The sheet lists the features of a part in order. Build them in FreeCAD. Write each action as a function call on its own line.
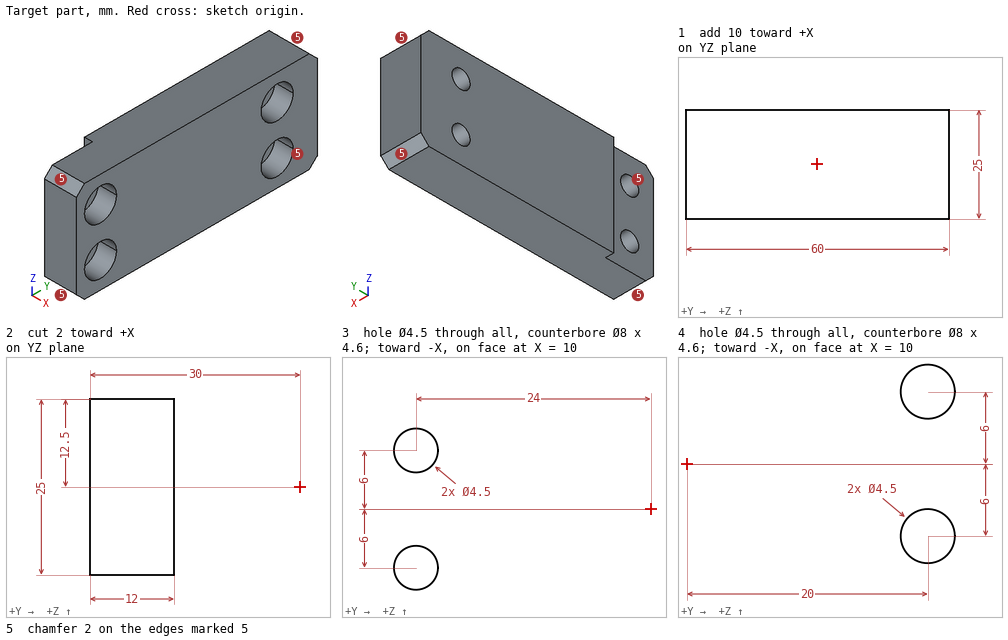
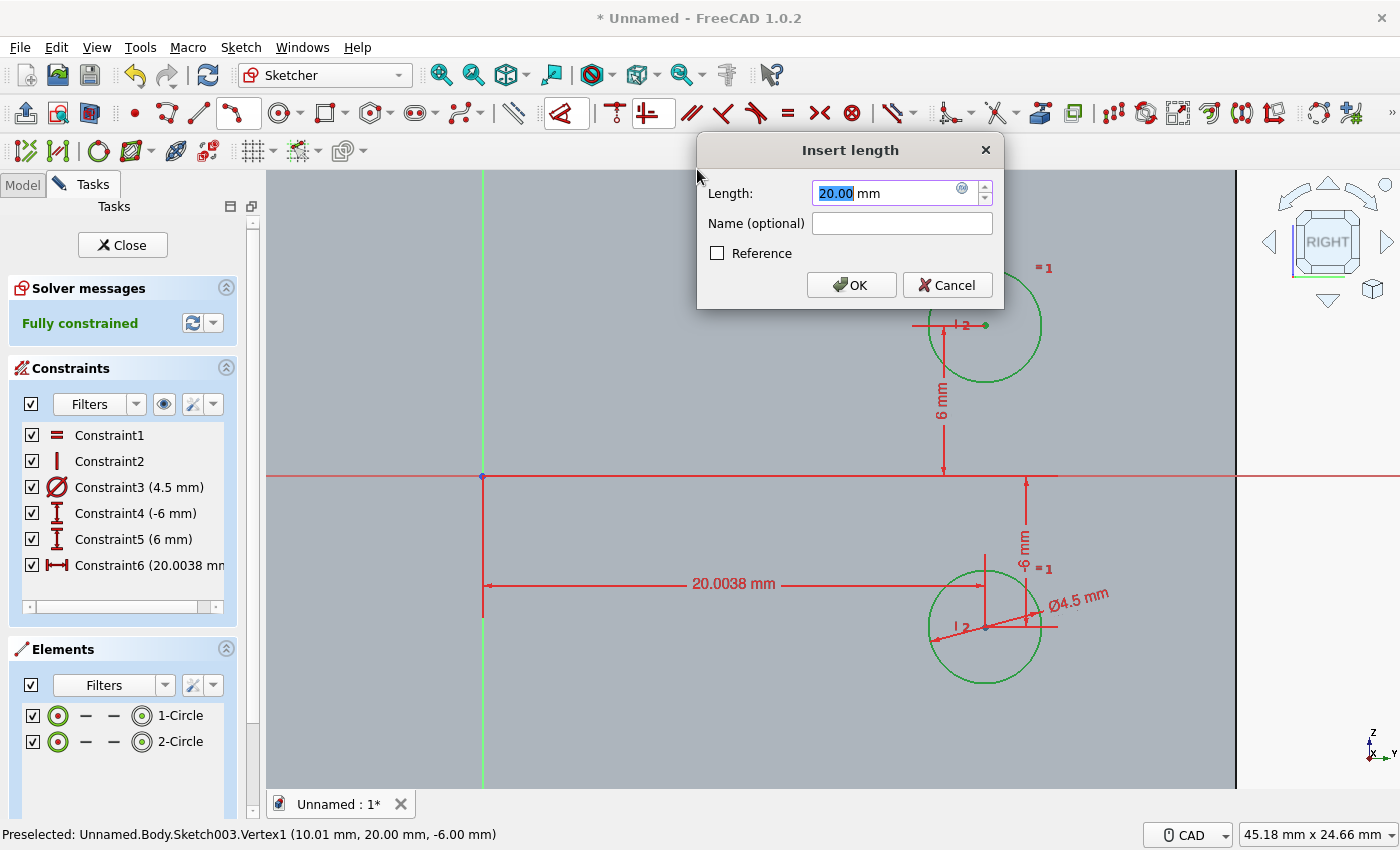
text(20)
key(Return)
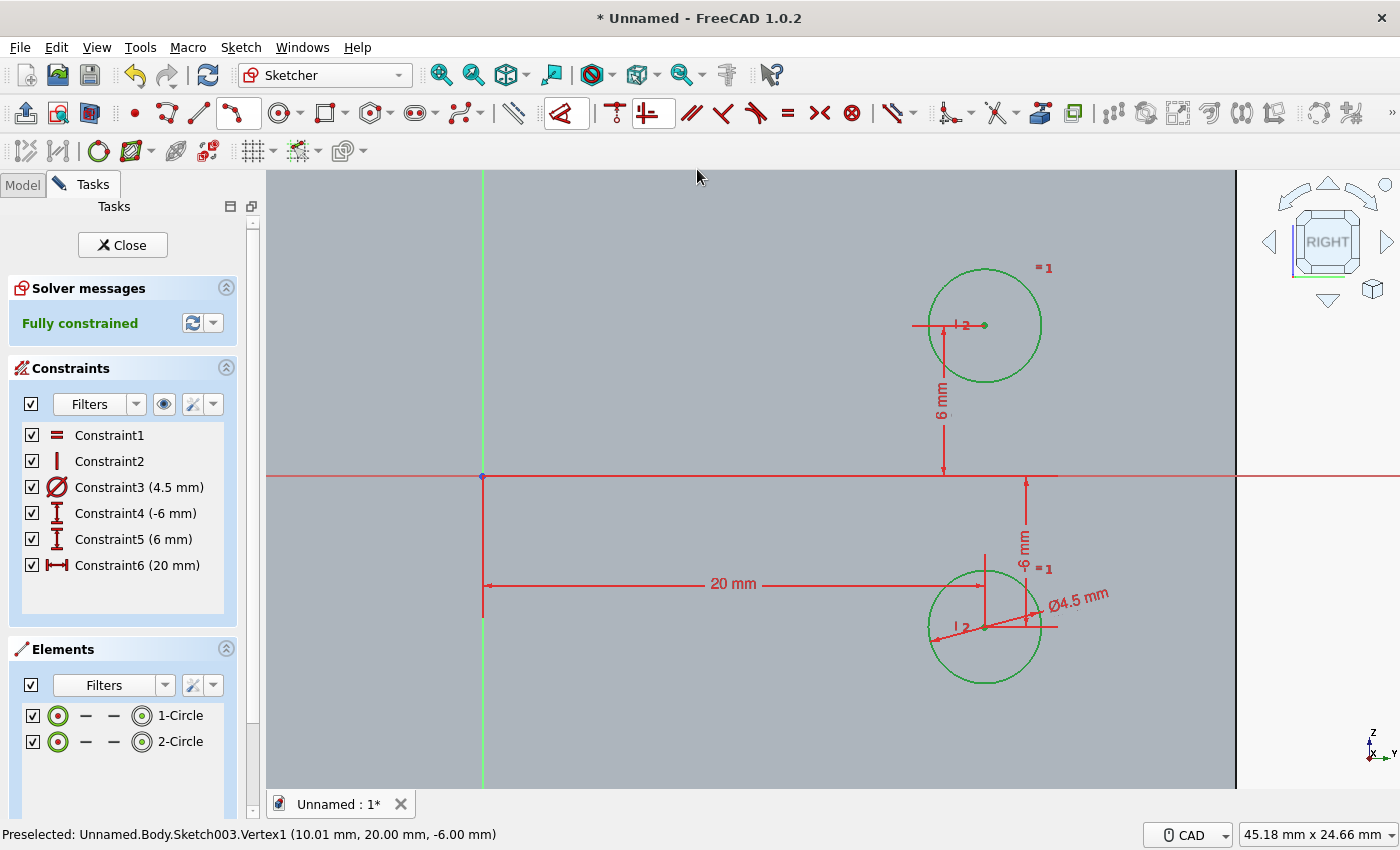
click(123, 245)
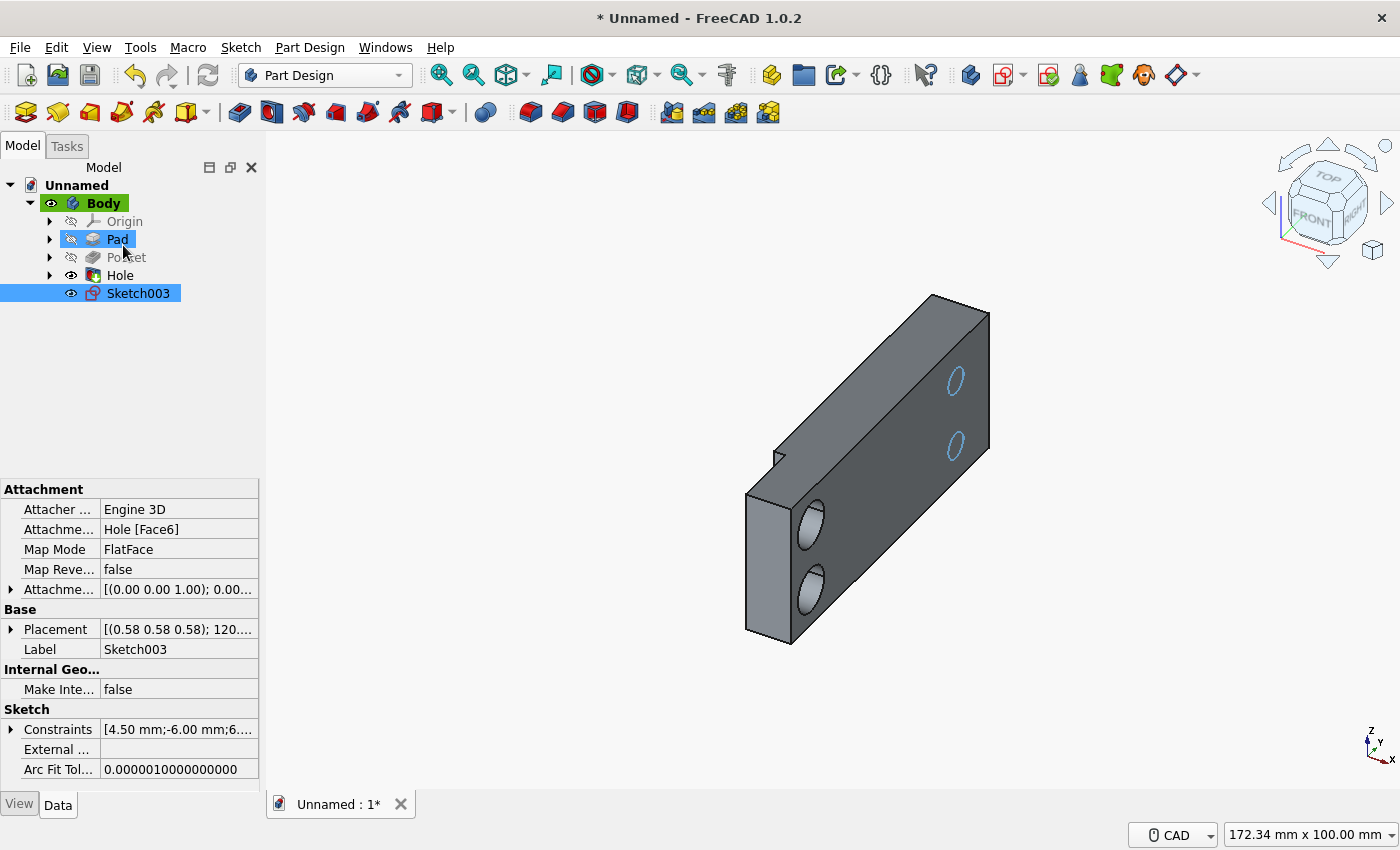
click(272, 112)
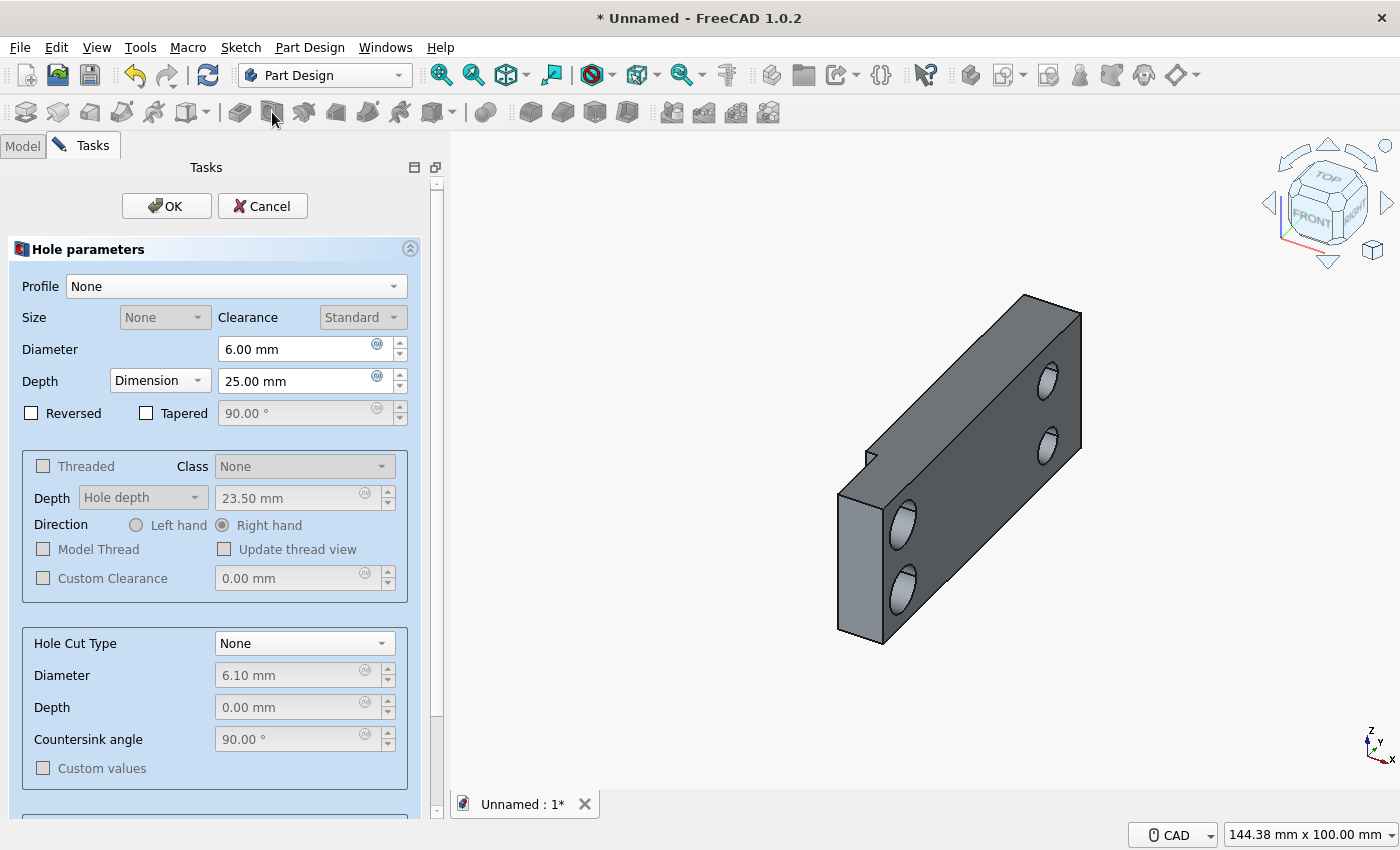
triple_click(305, 349)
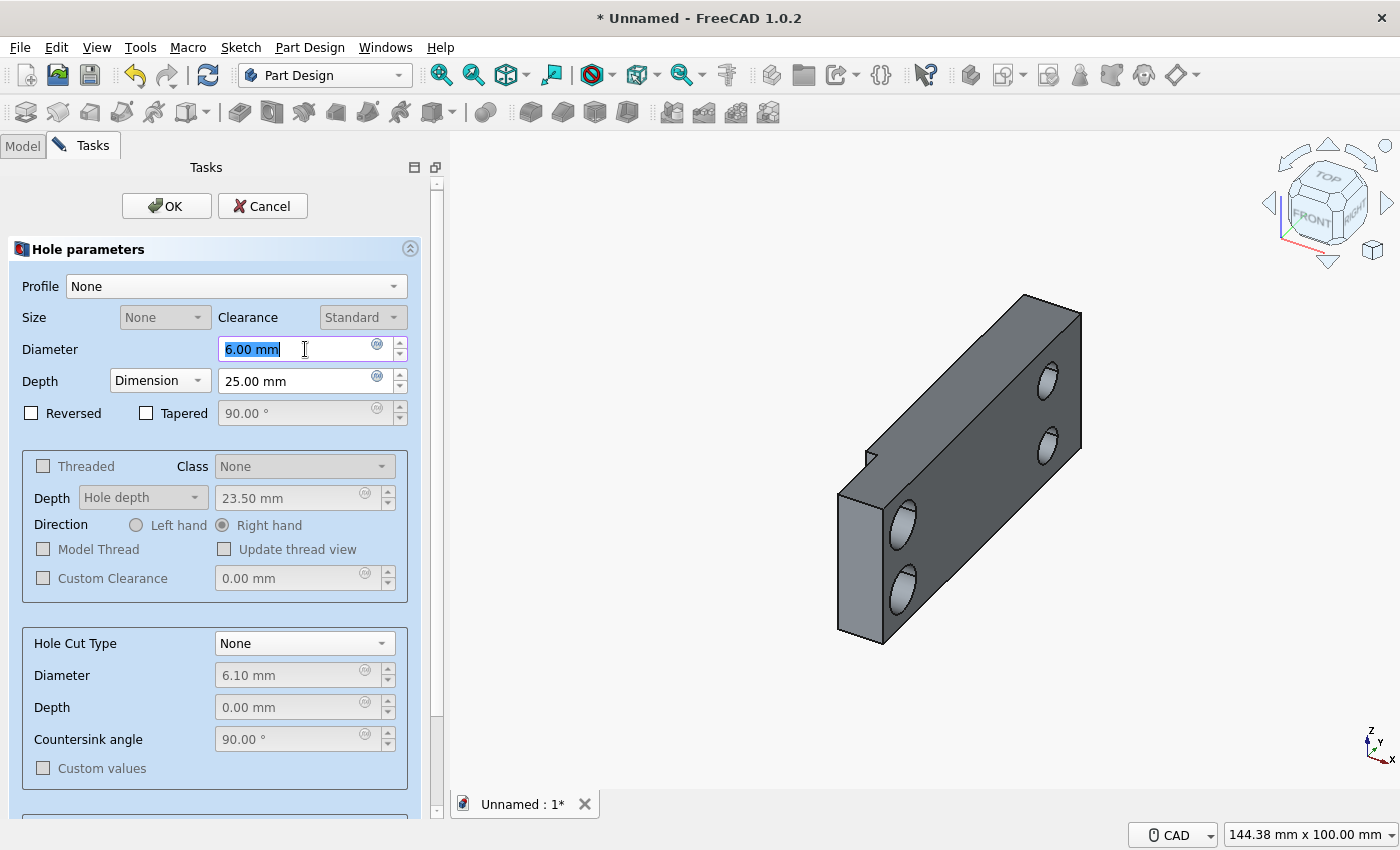
text(4.5)
key(Tab)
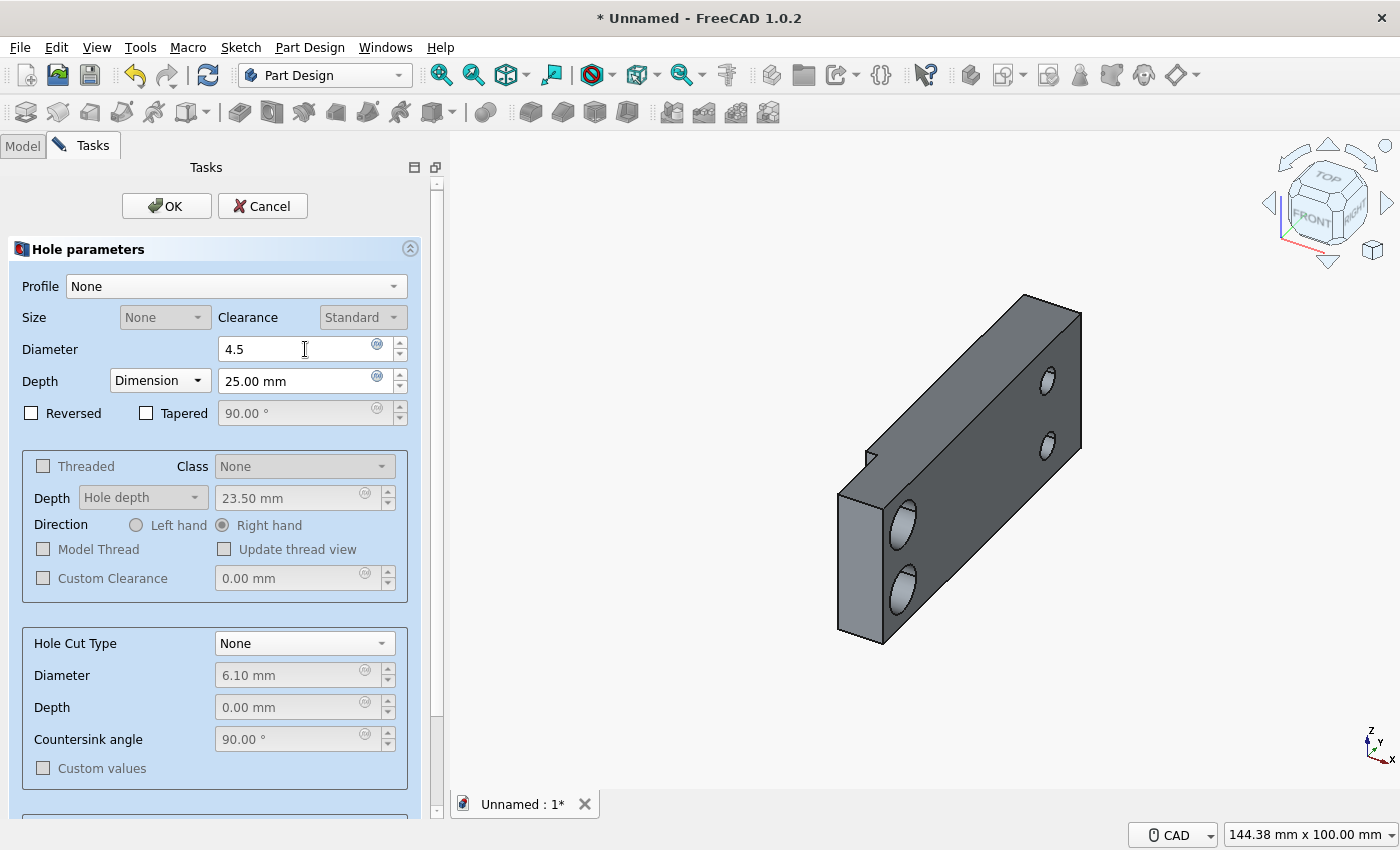
click(161, 380)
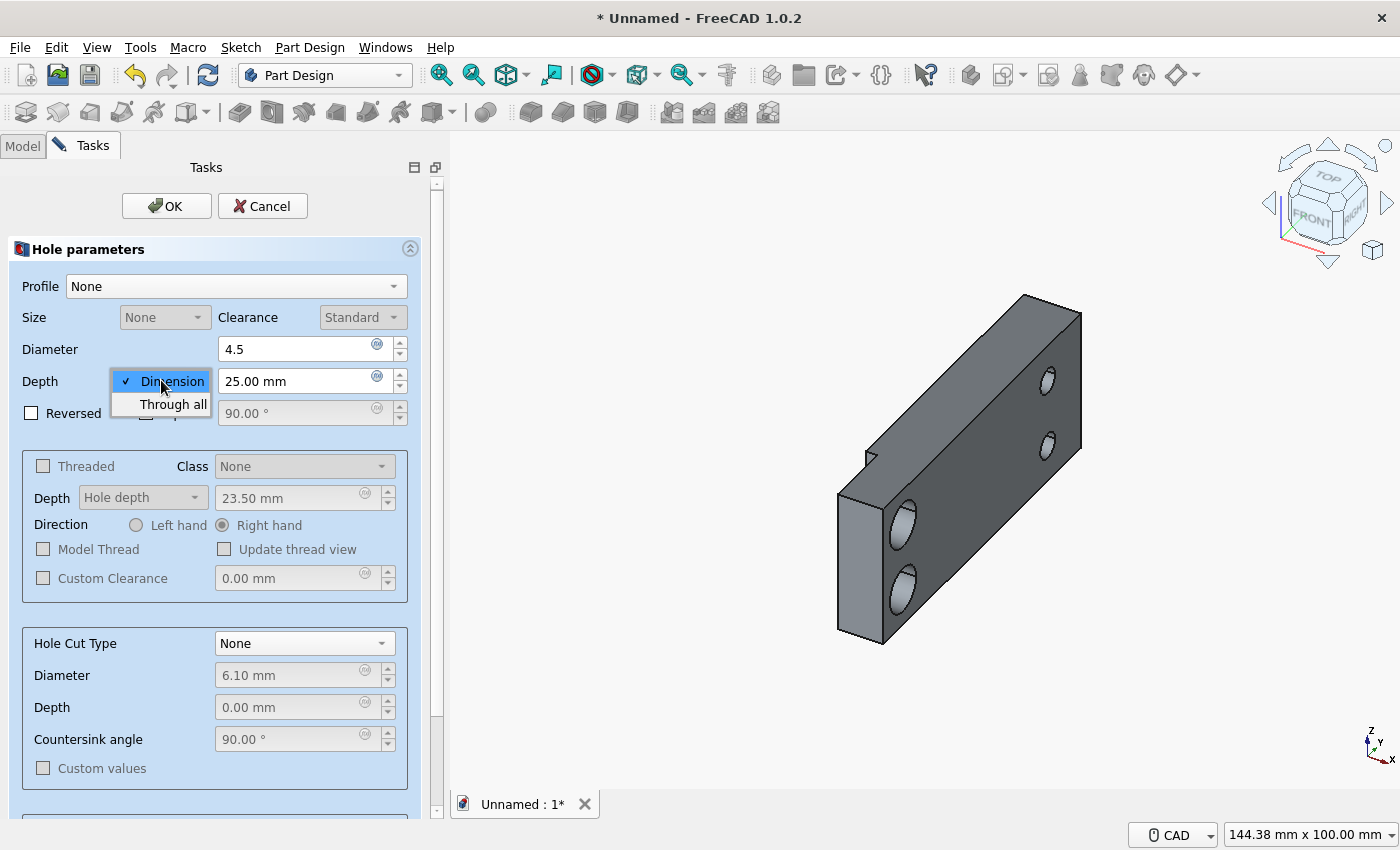
click(160, 404)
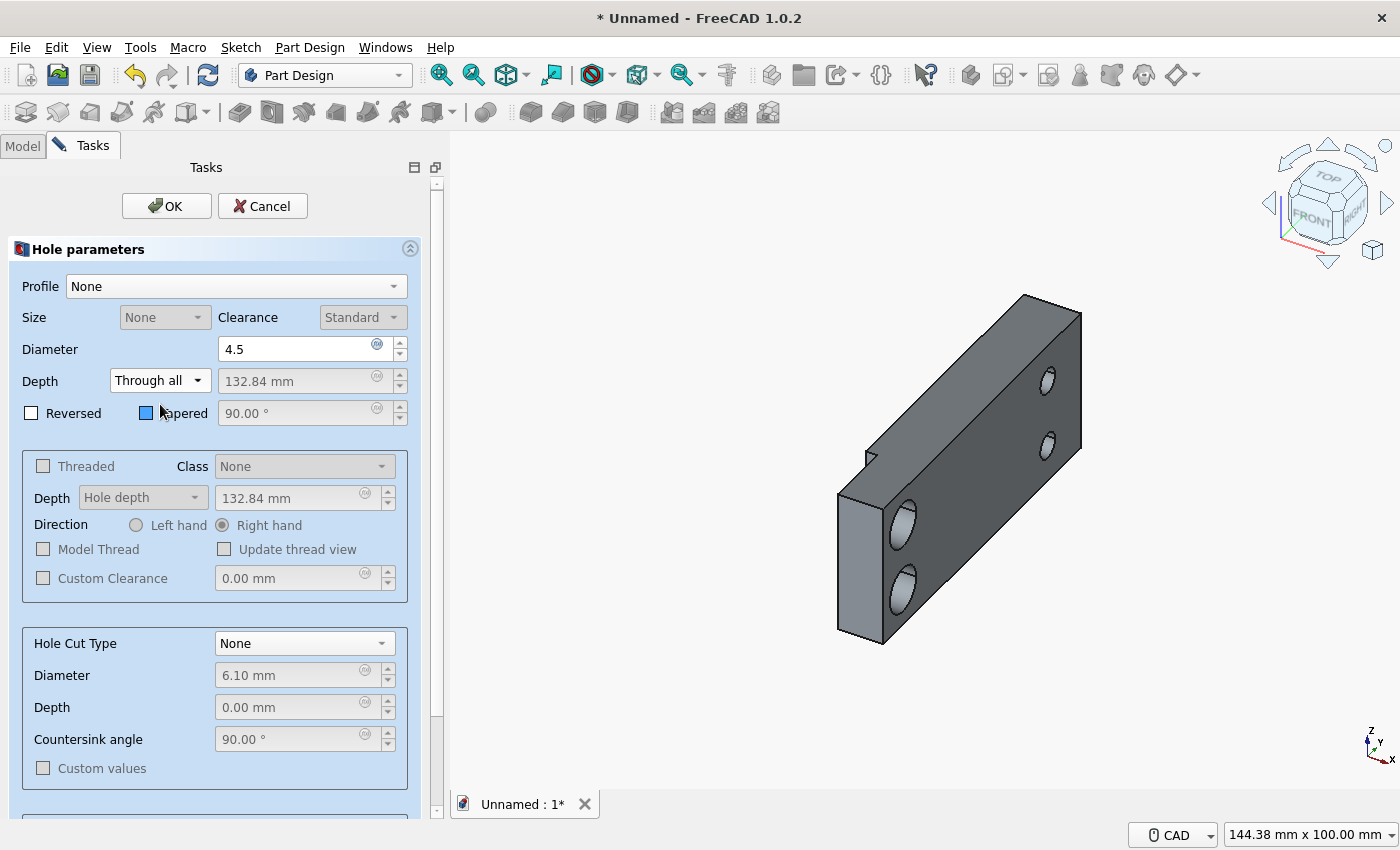
click(306, 644)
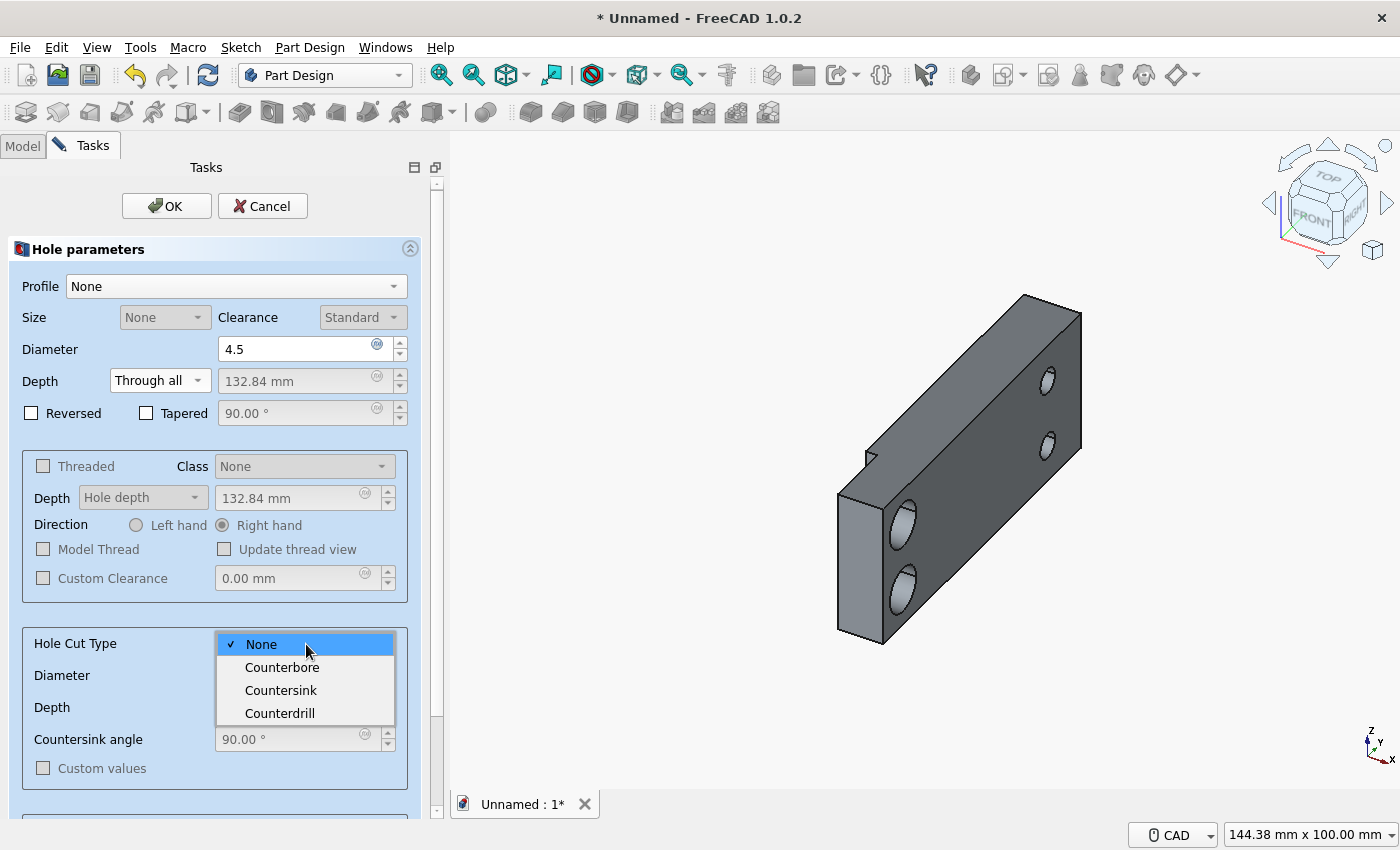
click(304, 668)